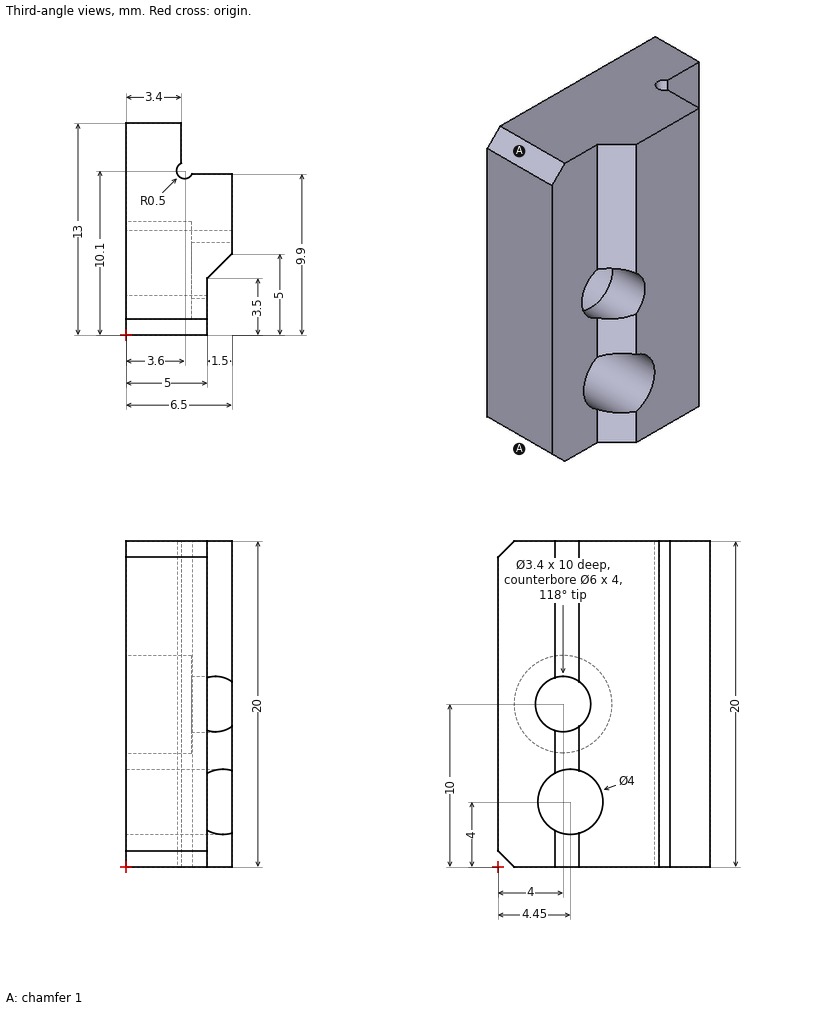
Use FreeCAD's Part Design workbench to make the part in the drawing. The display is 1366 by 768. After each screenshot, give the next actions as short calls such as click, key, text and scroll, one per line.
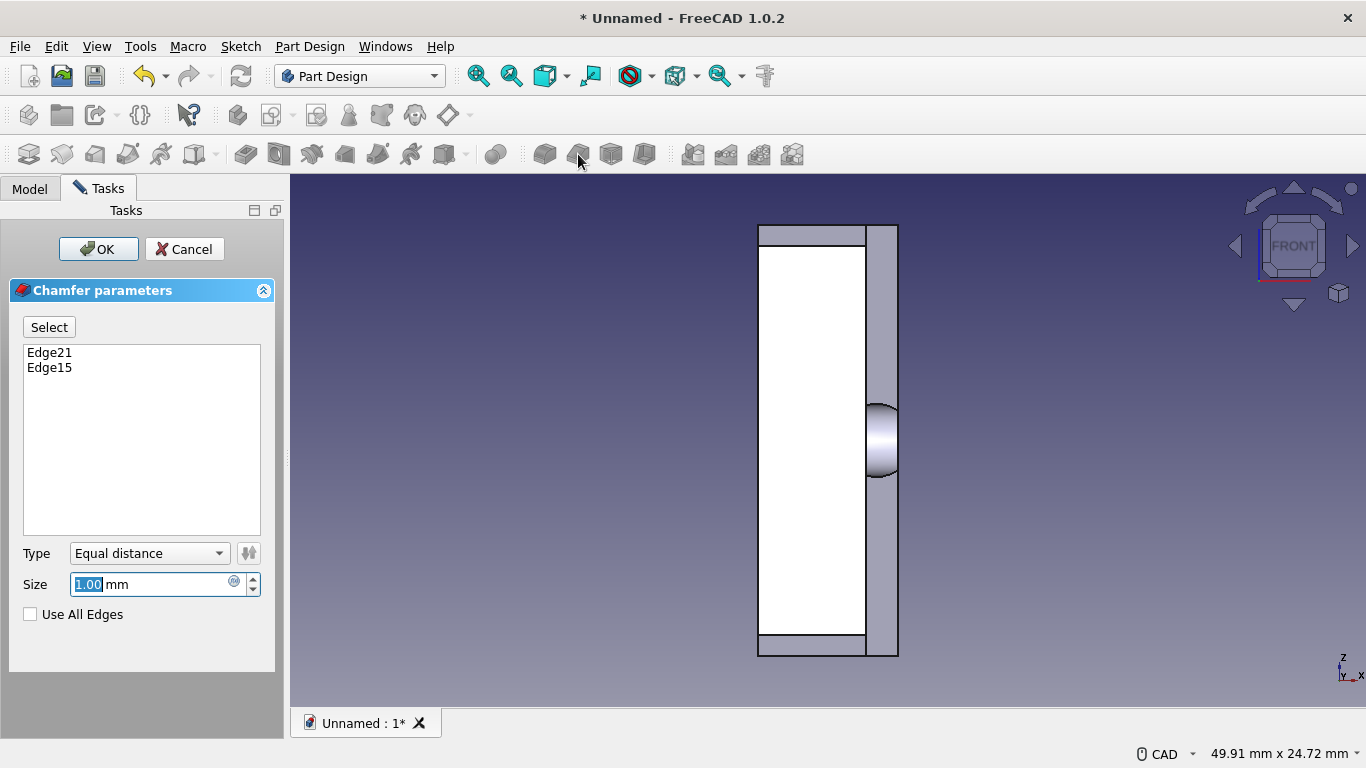
text(1)
key(Tab)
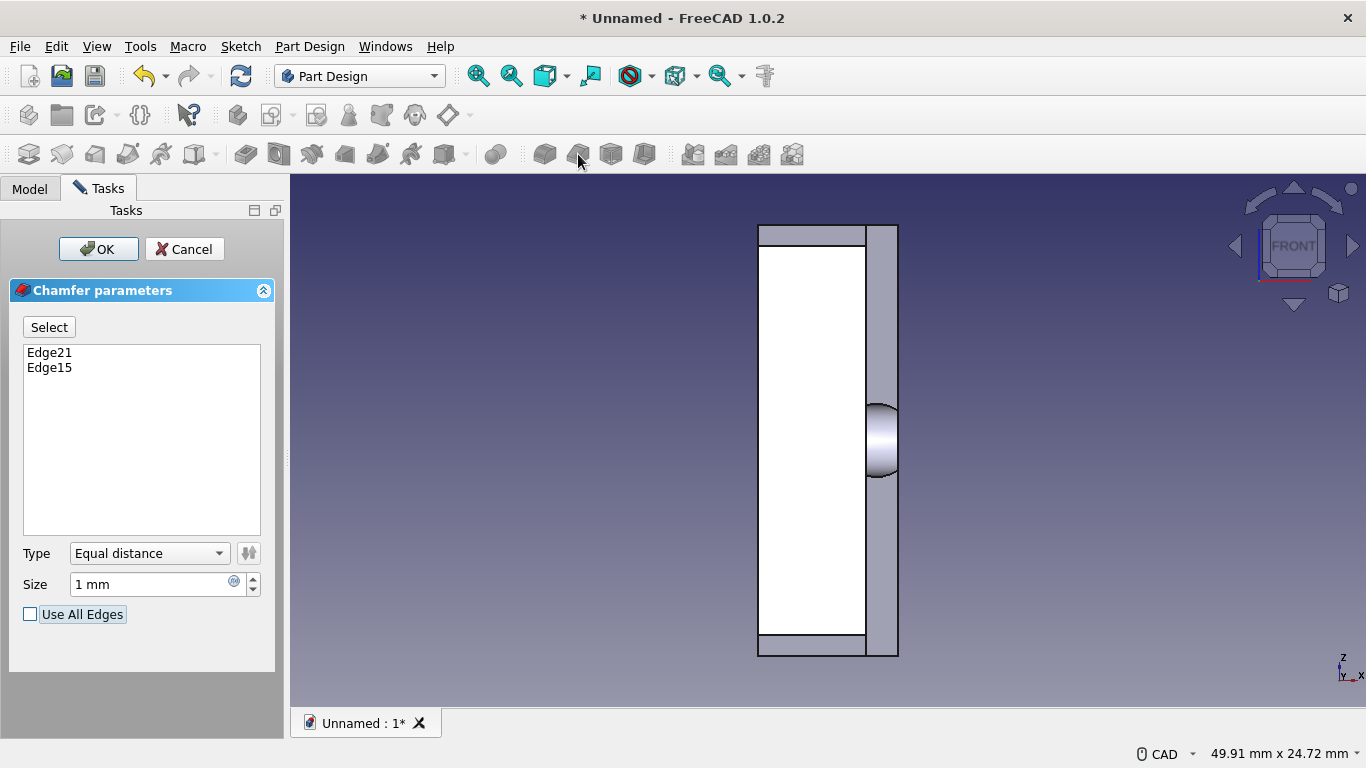
click(99, 249)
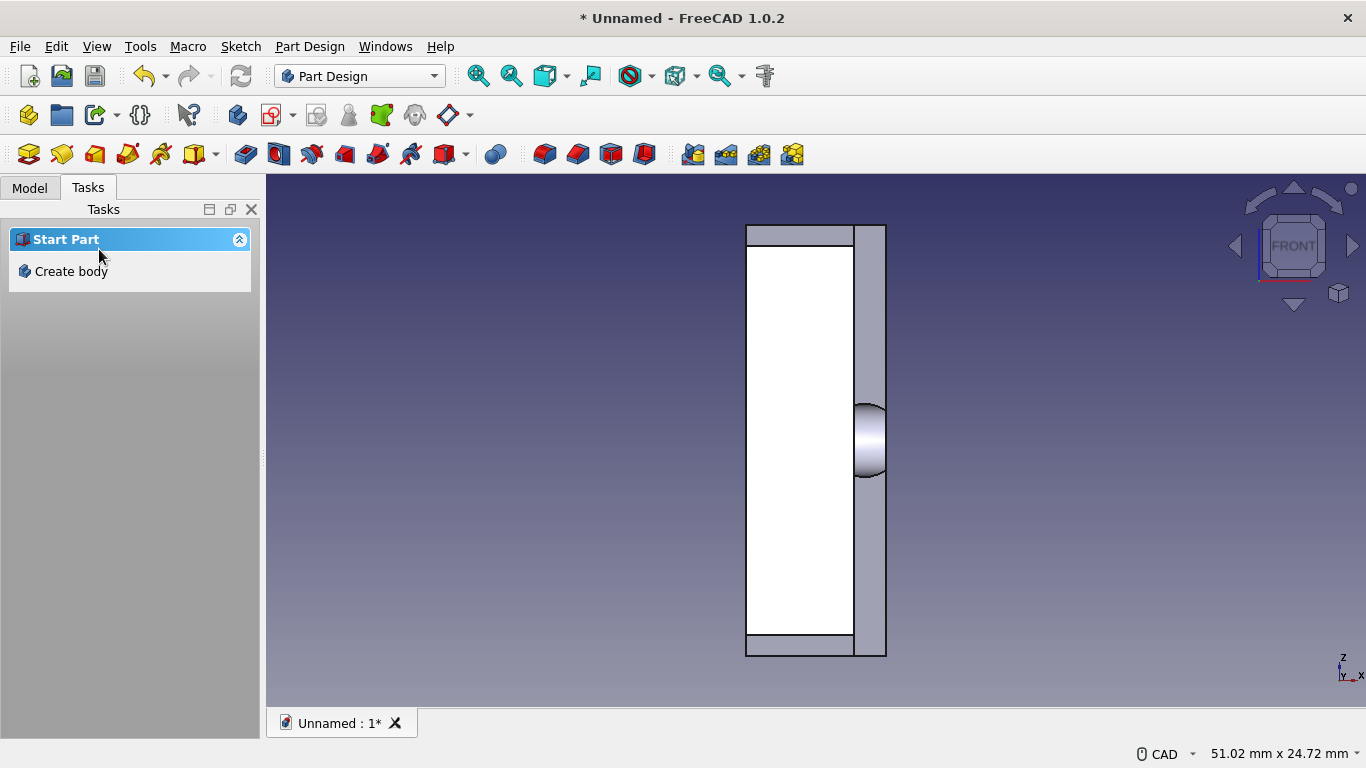
key(6)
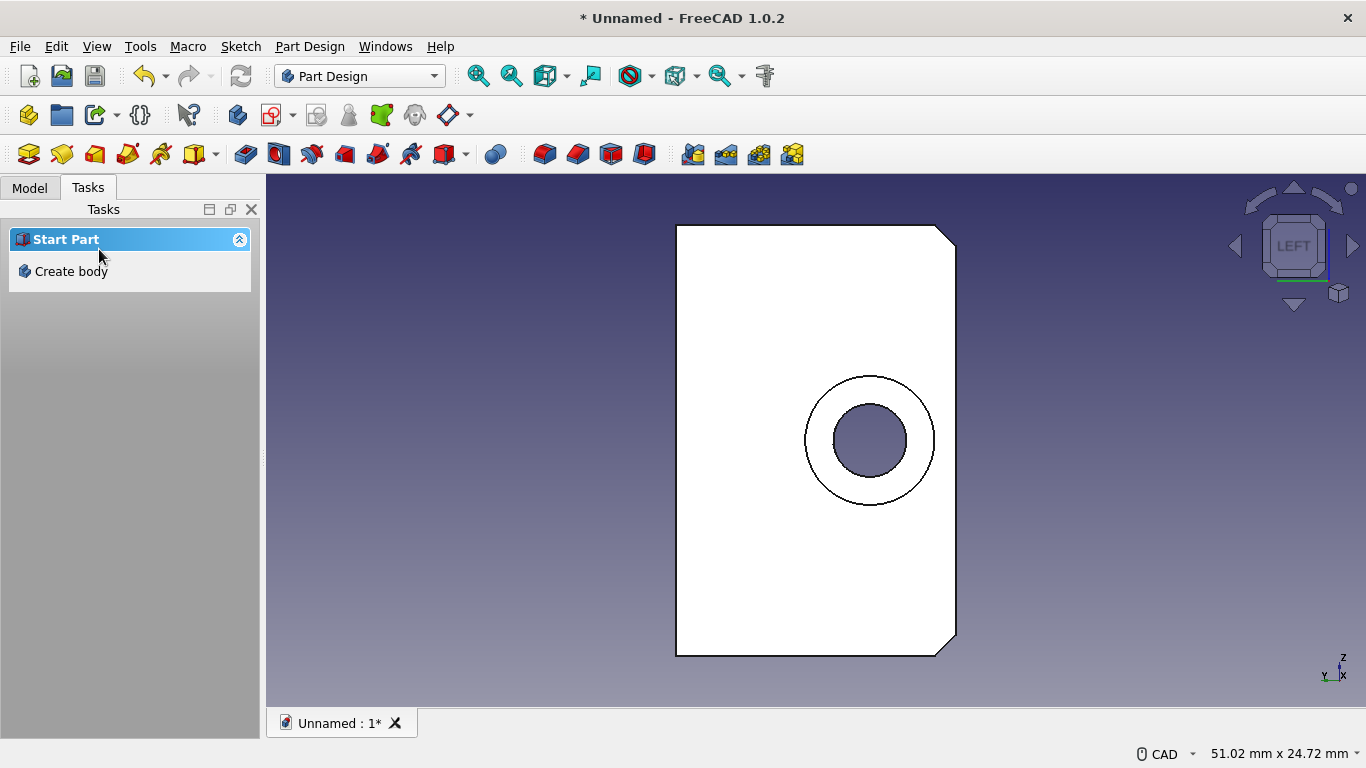
click(776, 316)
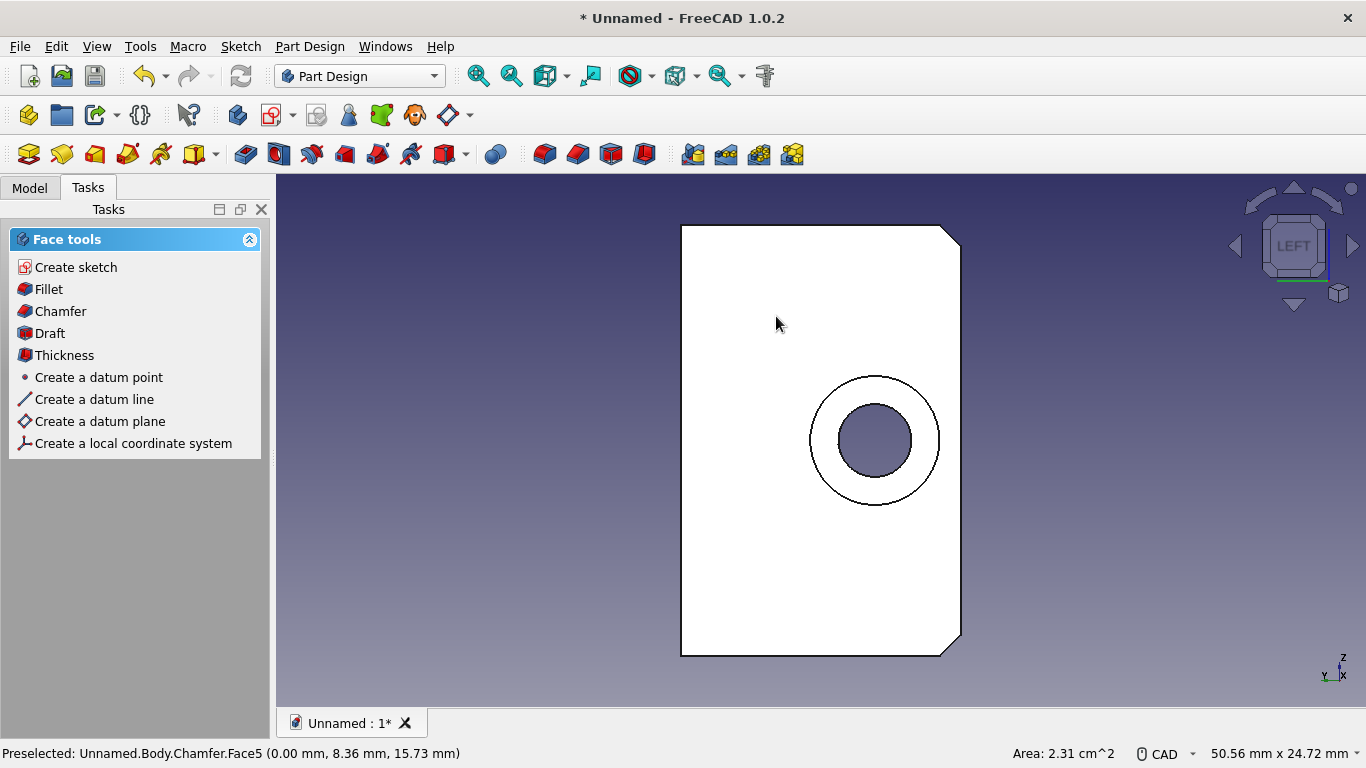
click(270, 116)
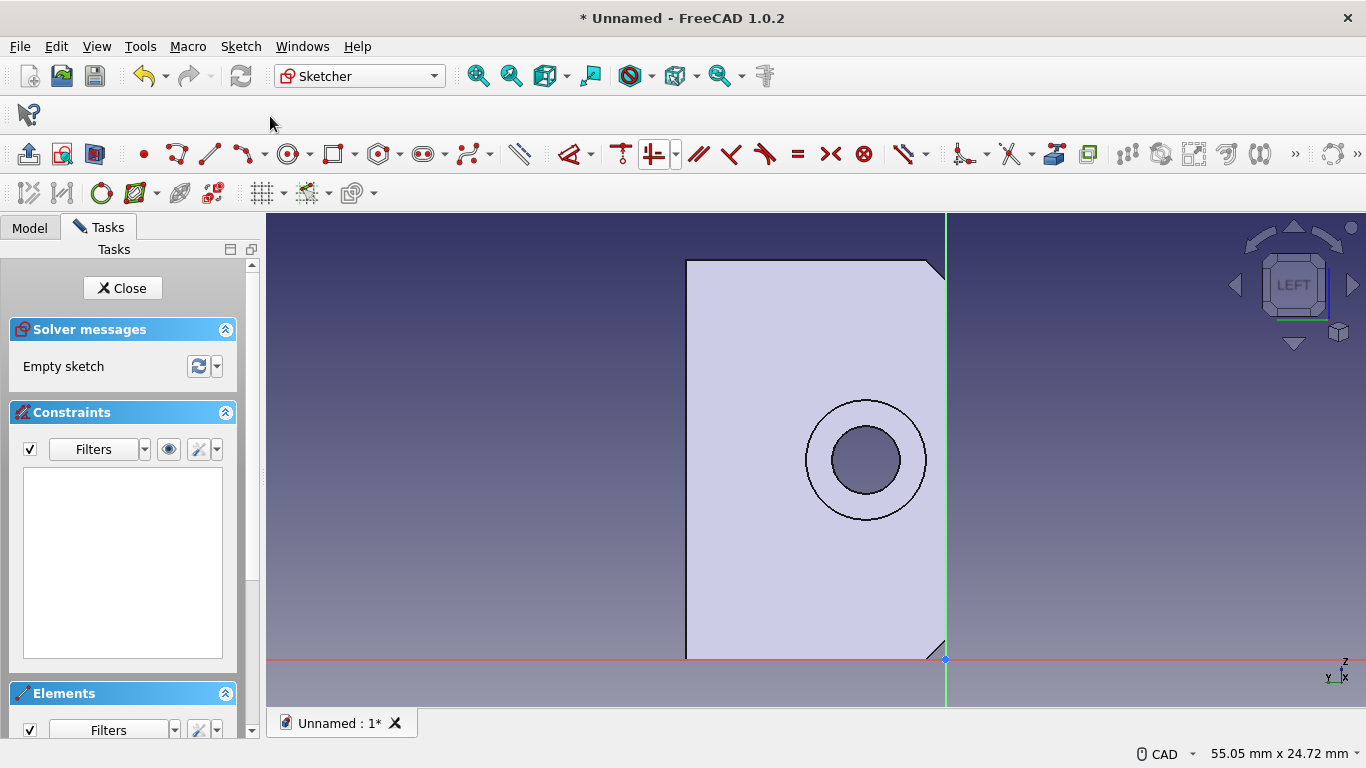
scroll(959, 679, up, 5)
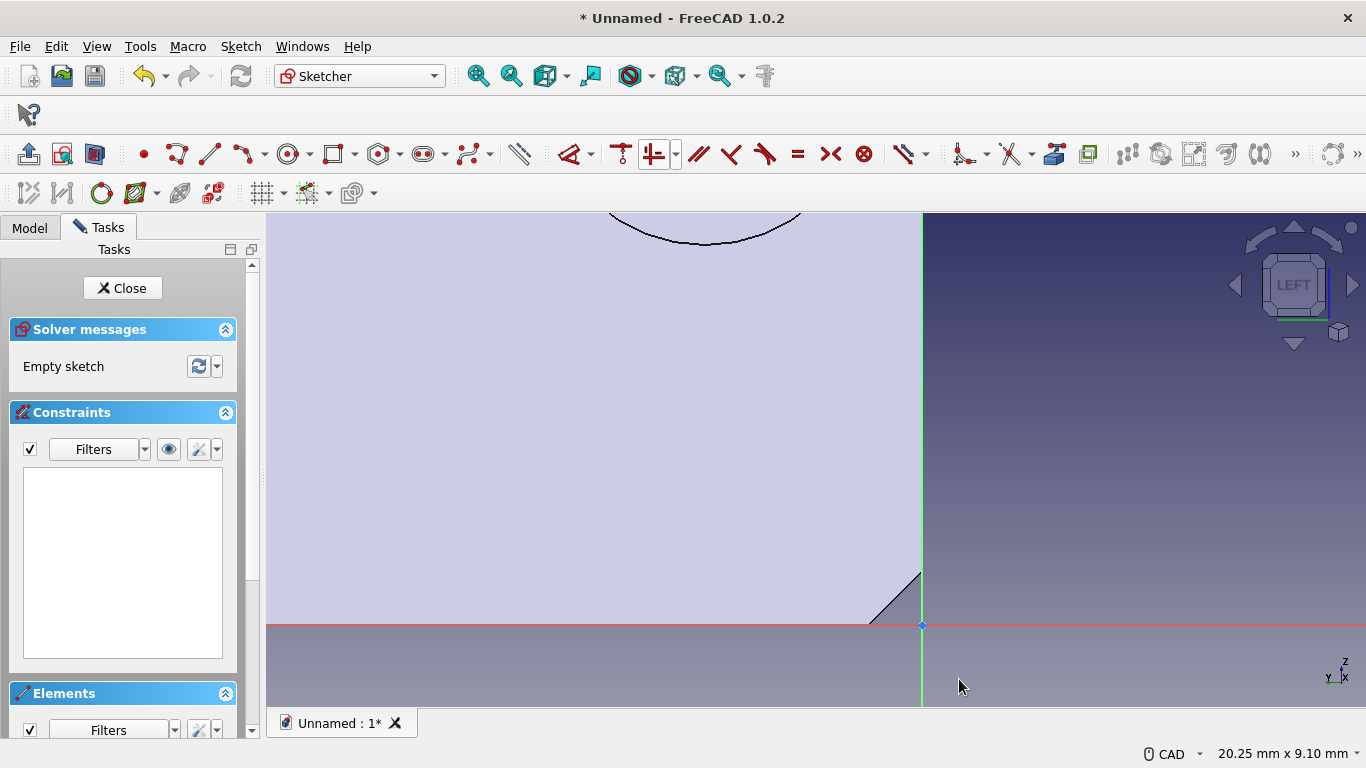
click(288, 154)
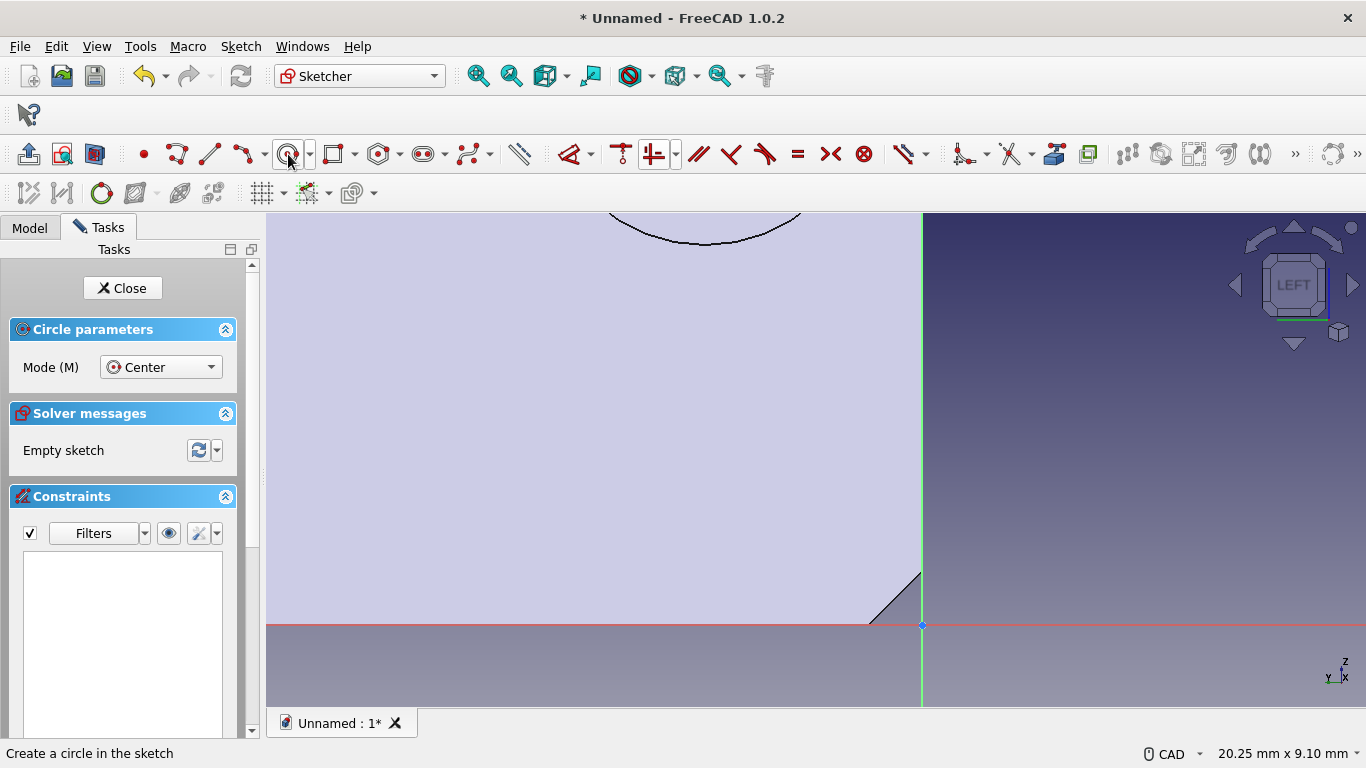
click(681, 408)
click(757, 331)
key(Escape)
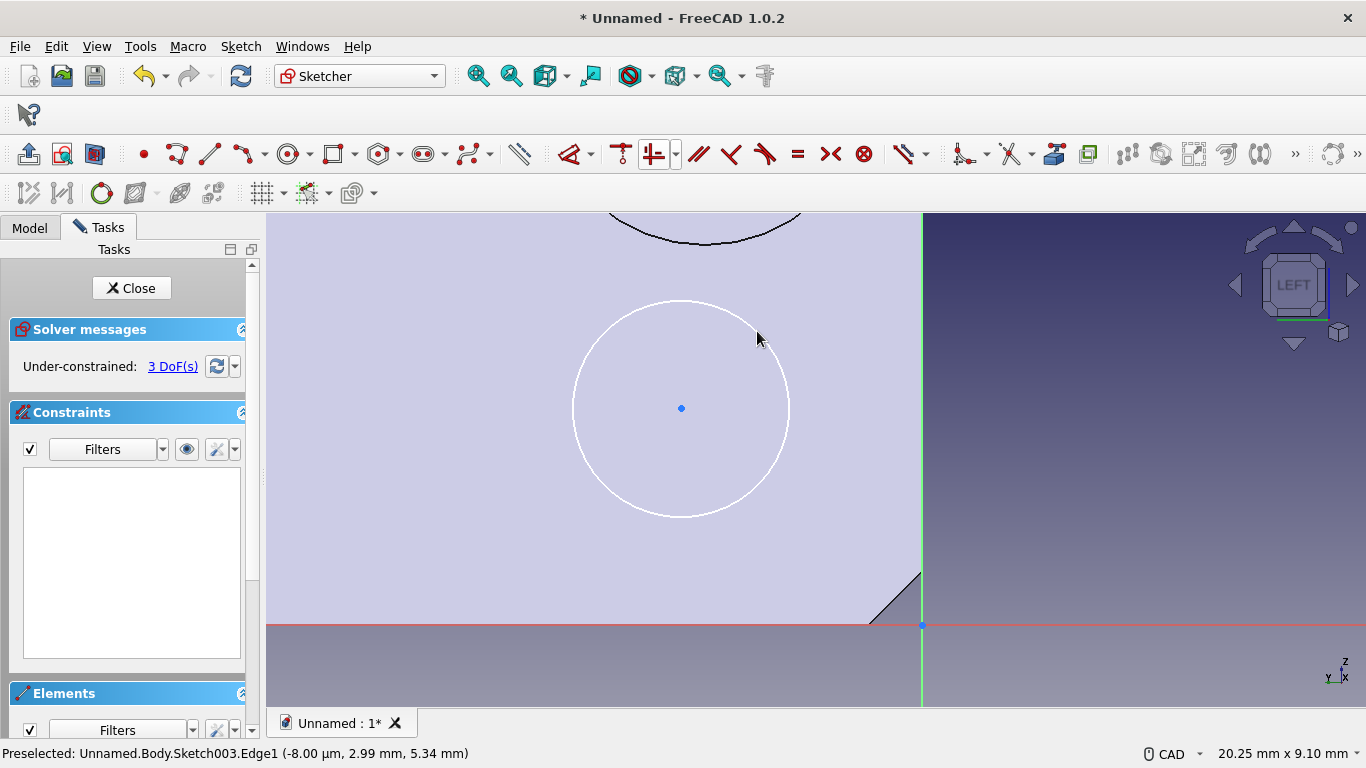
click(568, 154)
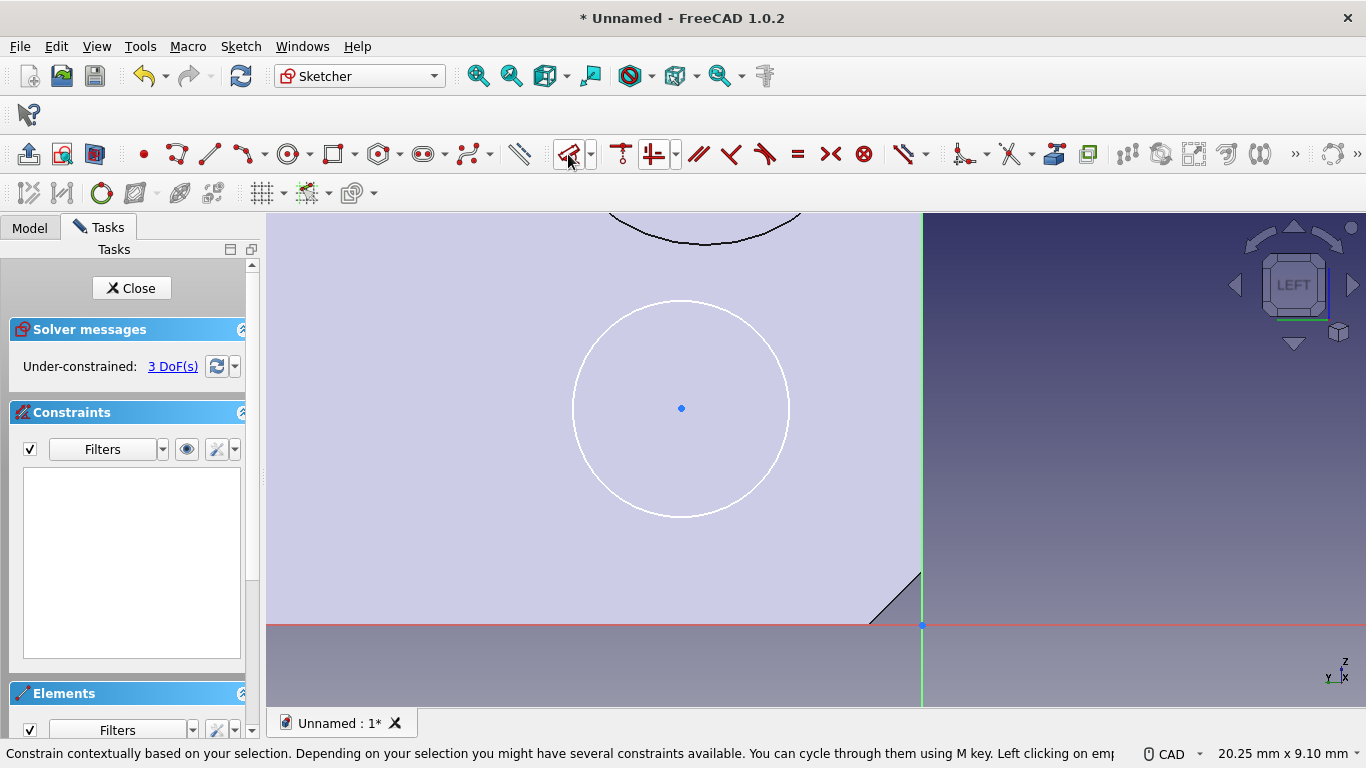
click(757, 332)
click(779, 309)